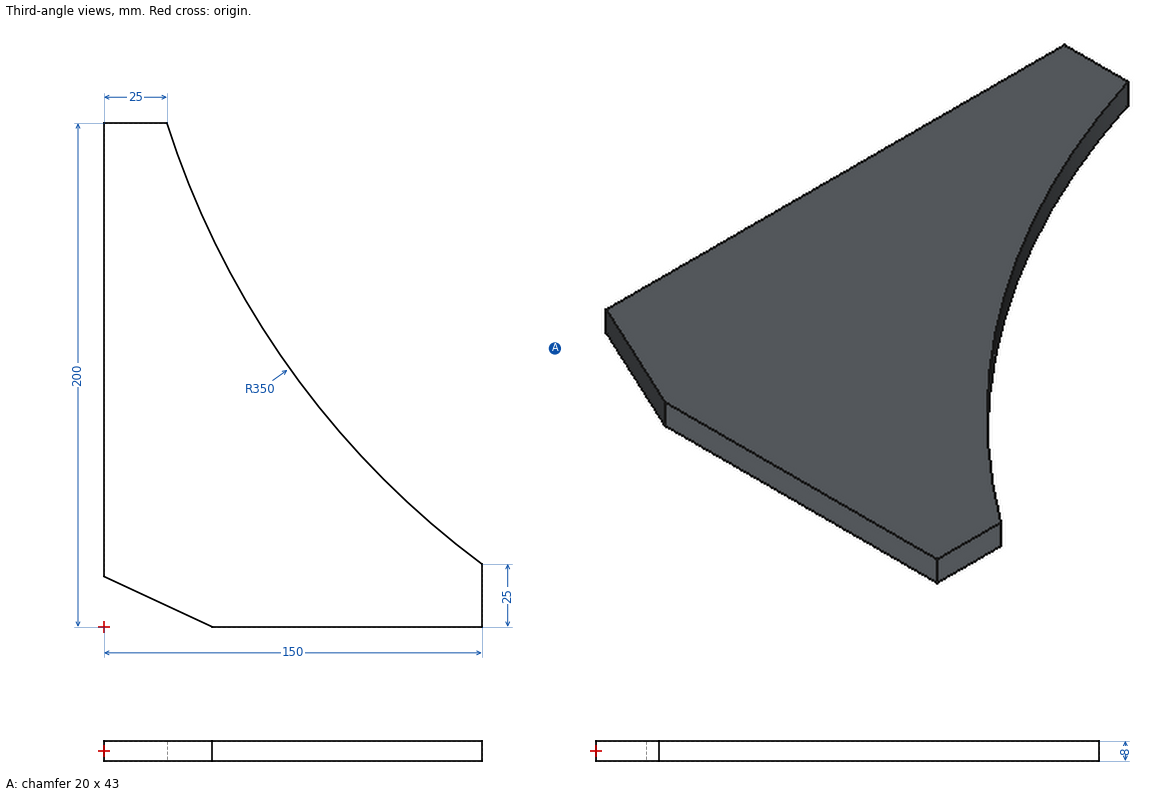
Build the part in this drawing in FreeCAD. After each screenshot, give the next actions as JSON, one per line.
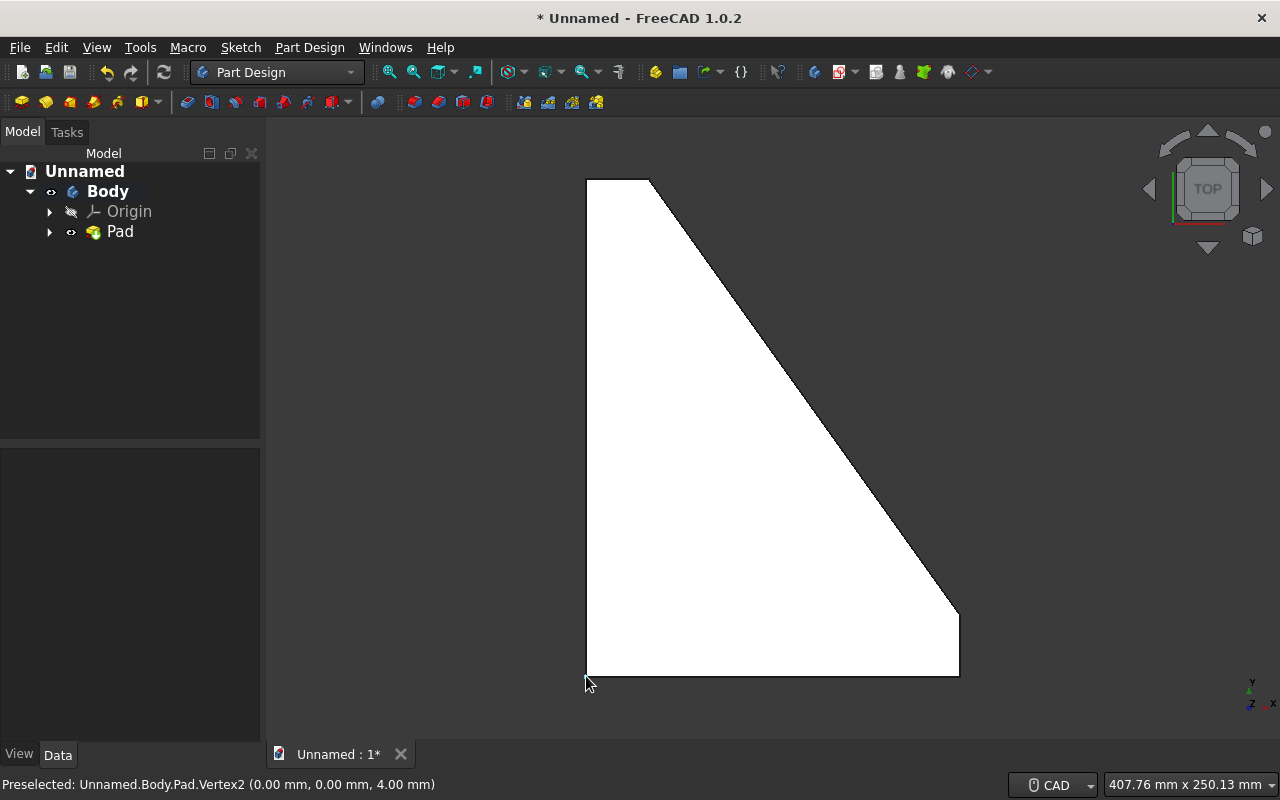
{"action": "key", "text": "1"}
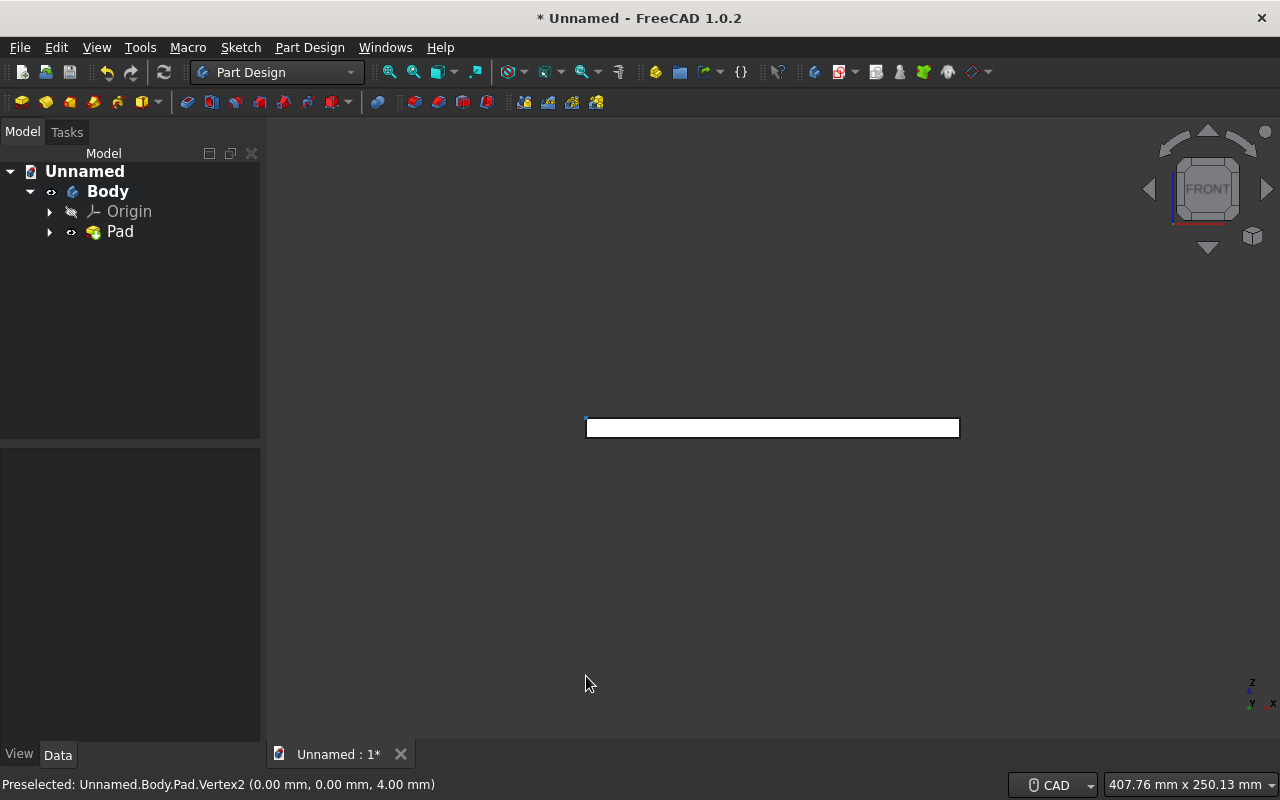
{"action": "left_click", "coordinate": [390, 72]}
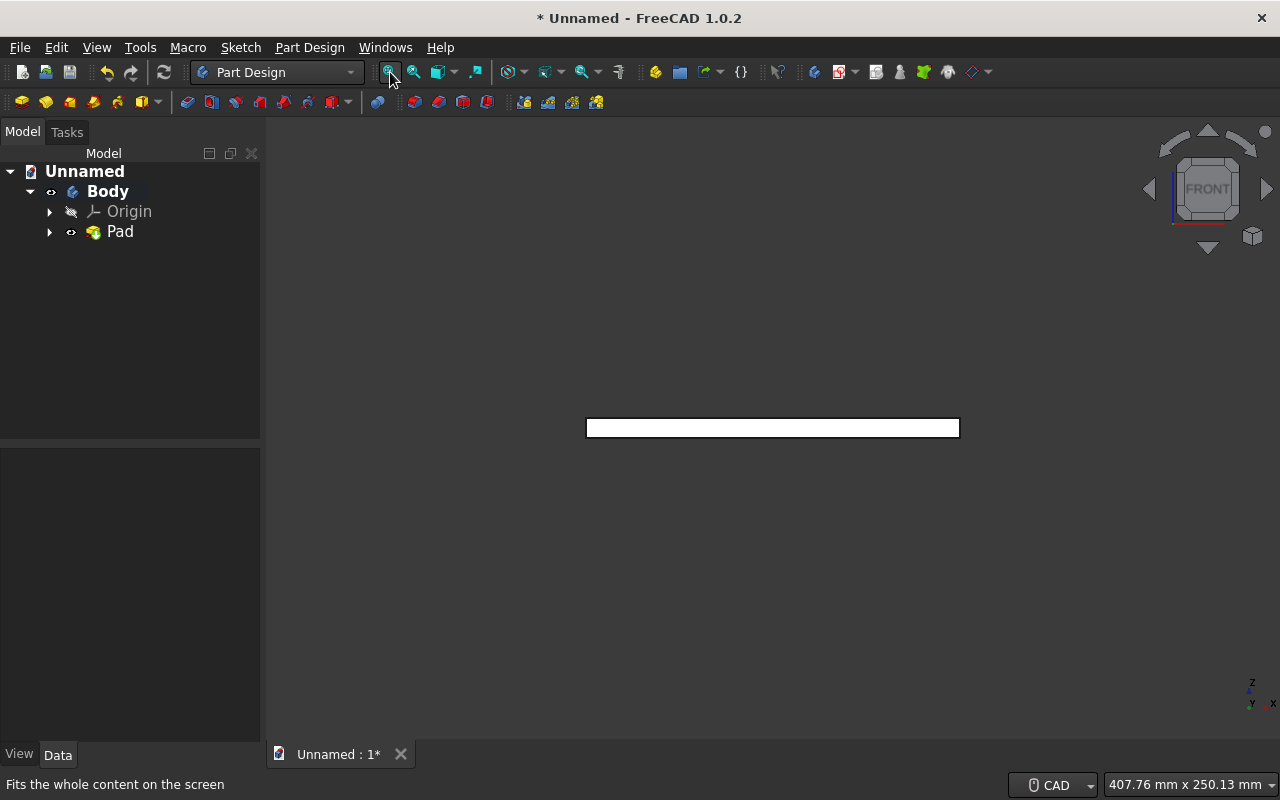
{"action": "left_click", "coordinate": [586, 427]}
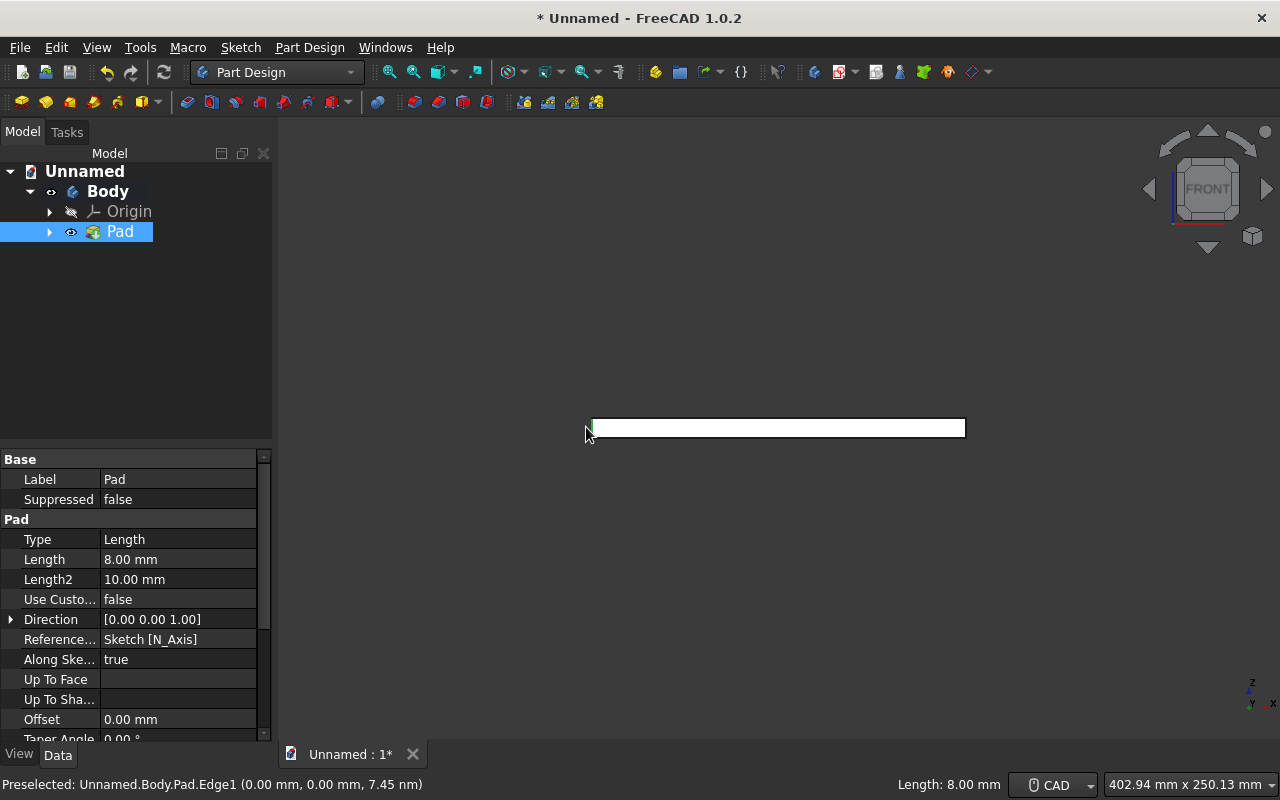
{"action": "left_click", "coordinate": [440, 102]}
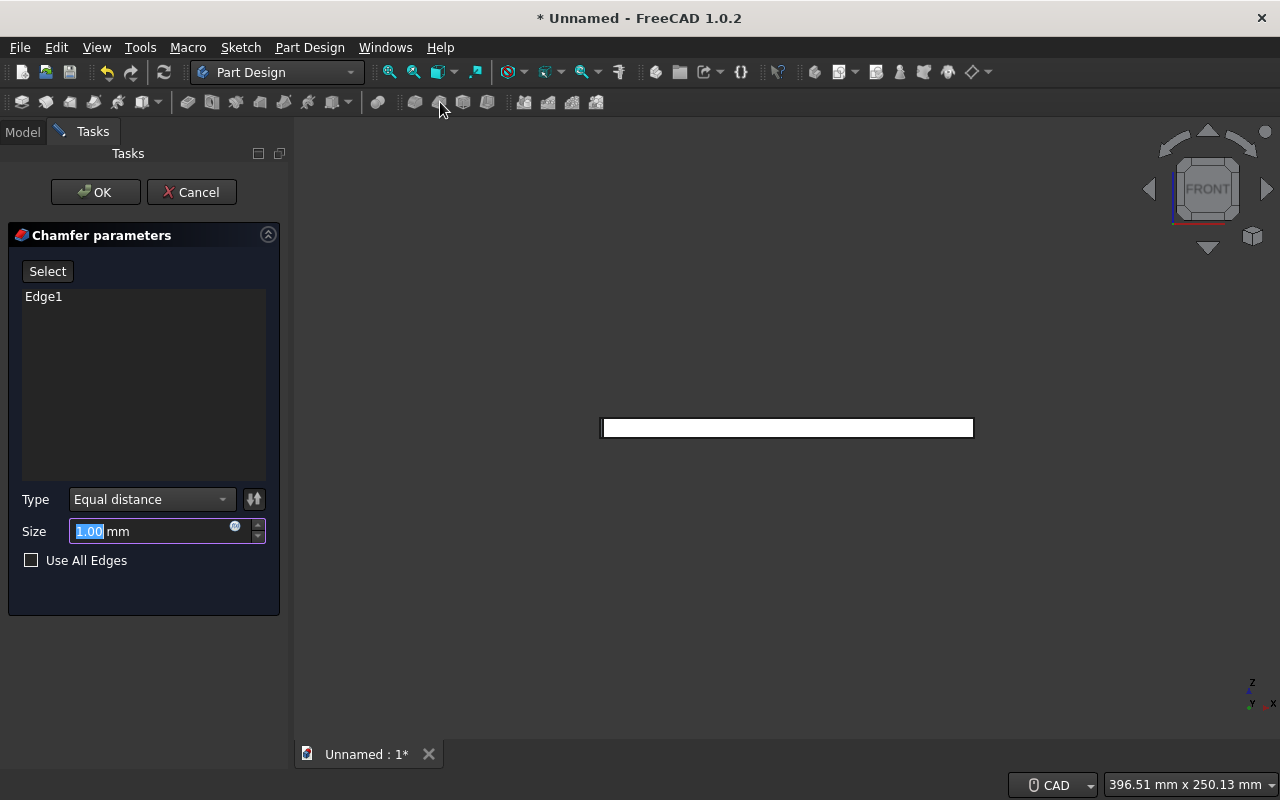
{"action": "type", "text": "20"}
{"action": "key", "text": "Tab"}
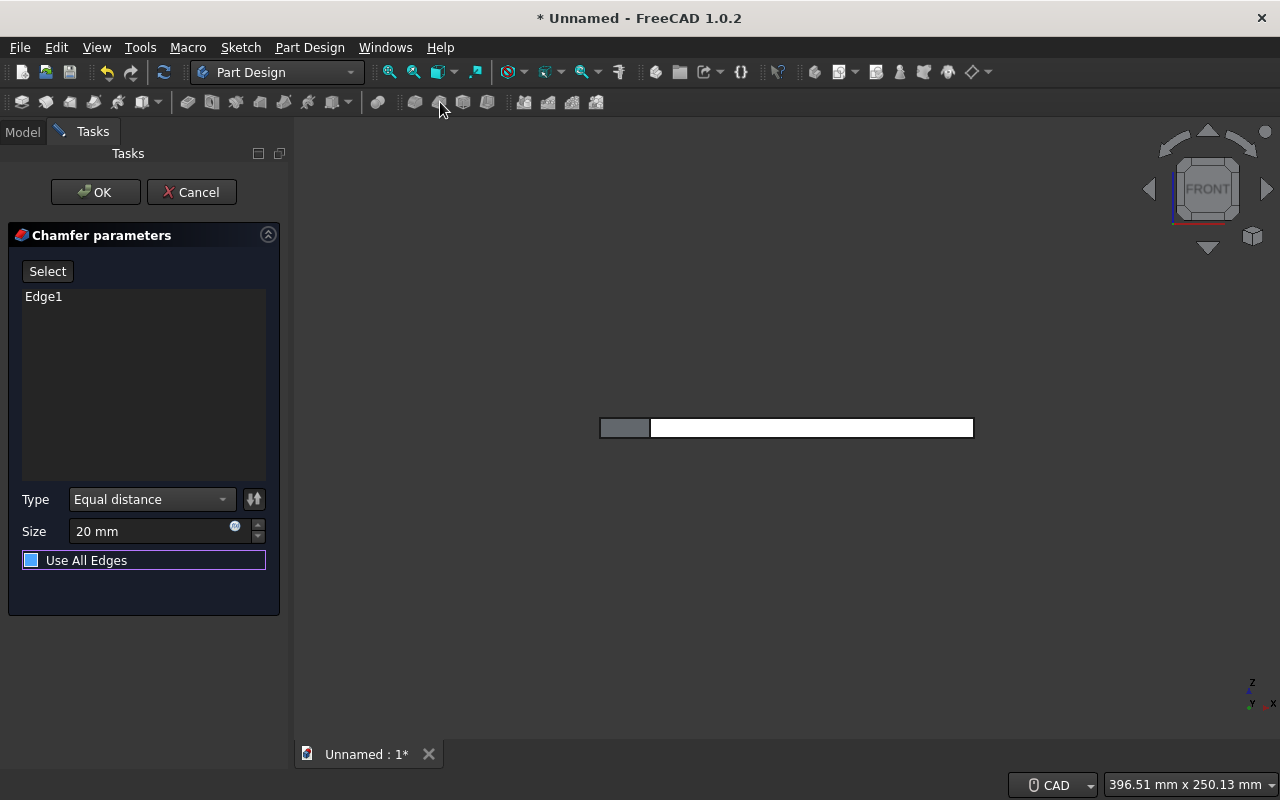
{"action": "left_click", "coordinate": [153, 500]}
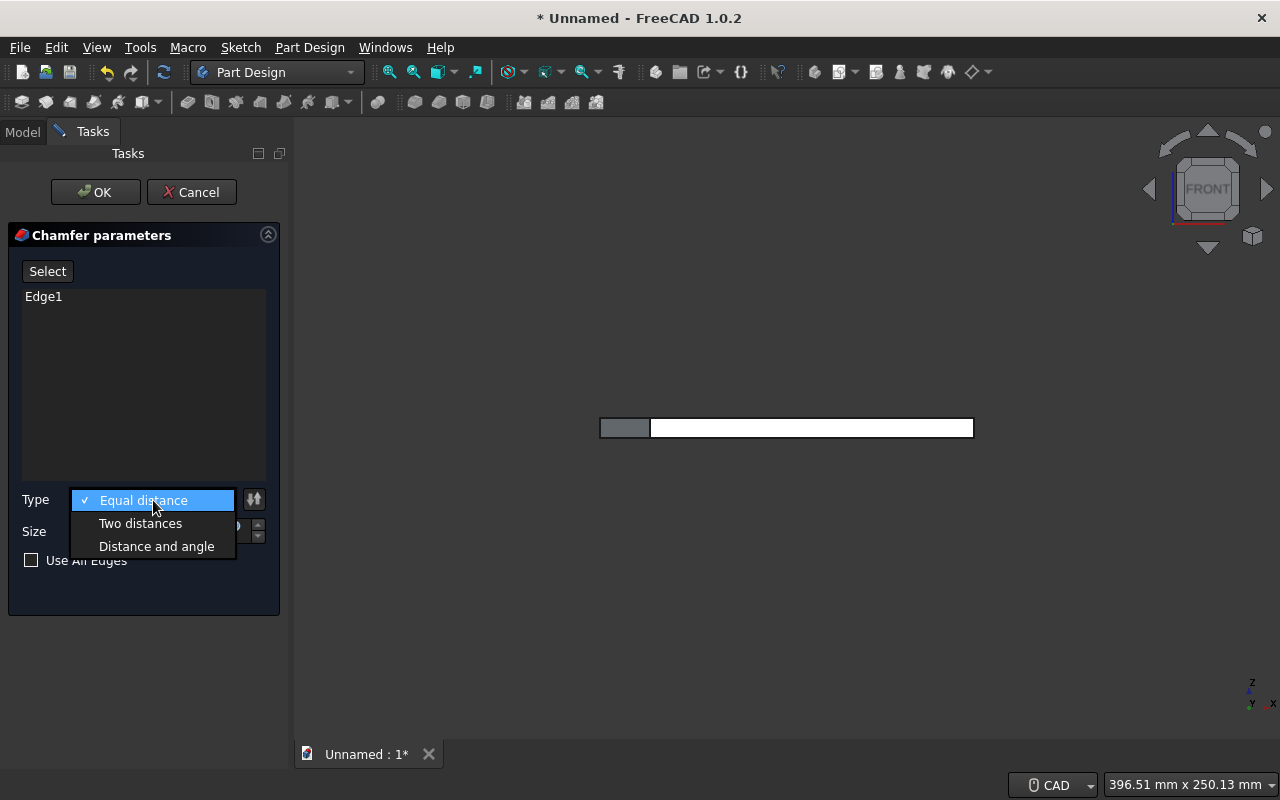
{"action": "left_click", "coordinate": [152, 524]}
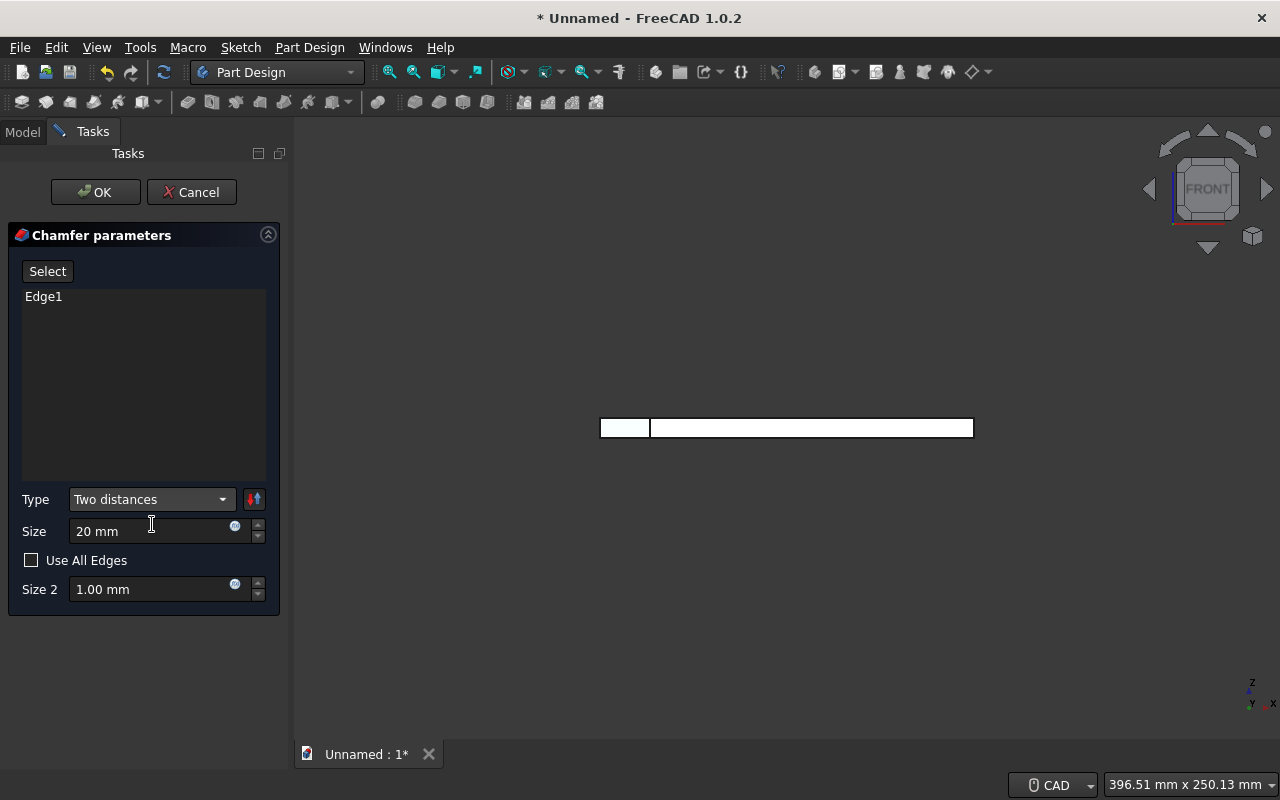
{"action": "triple_click", "coordinate": [160, 589]}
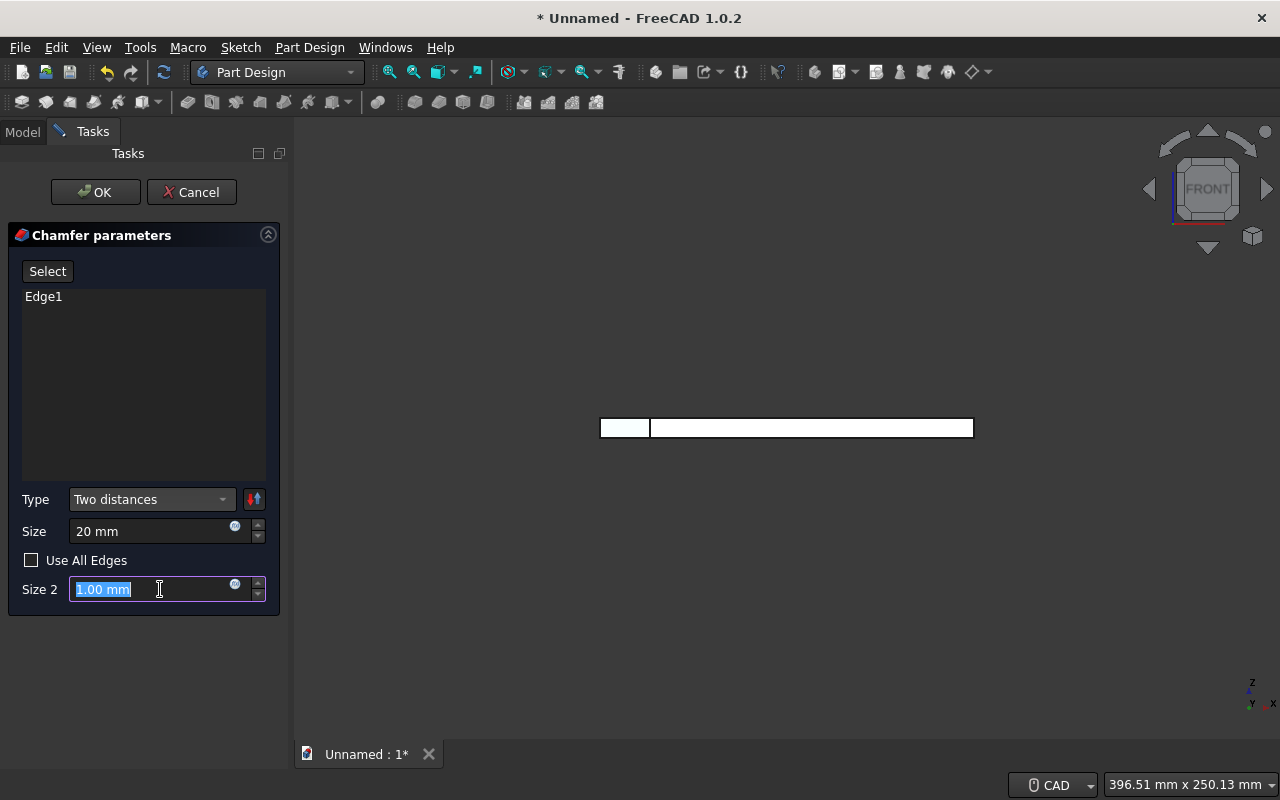
{"action": "type", "text": "43"}
{"action": "key", "text": "Tab"}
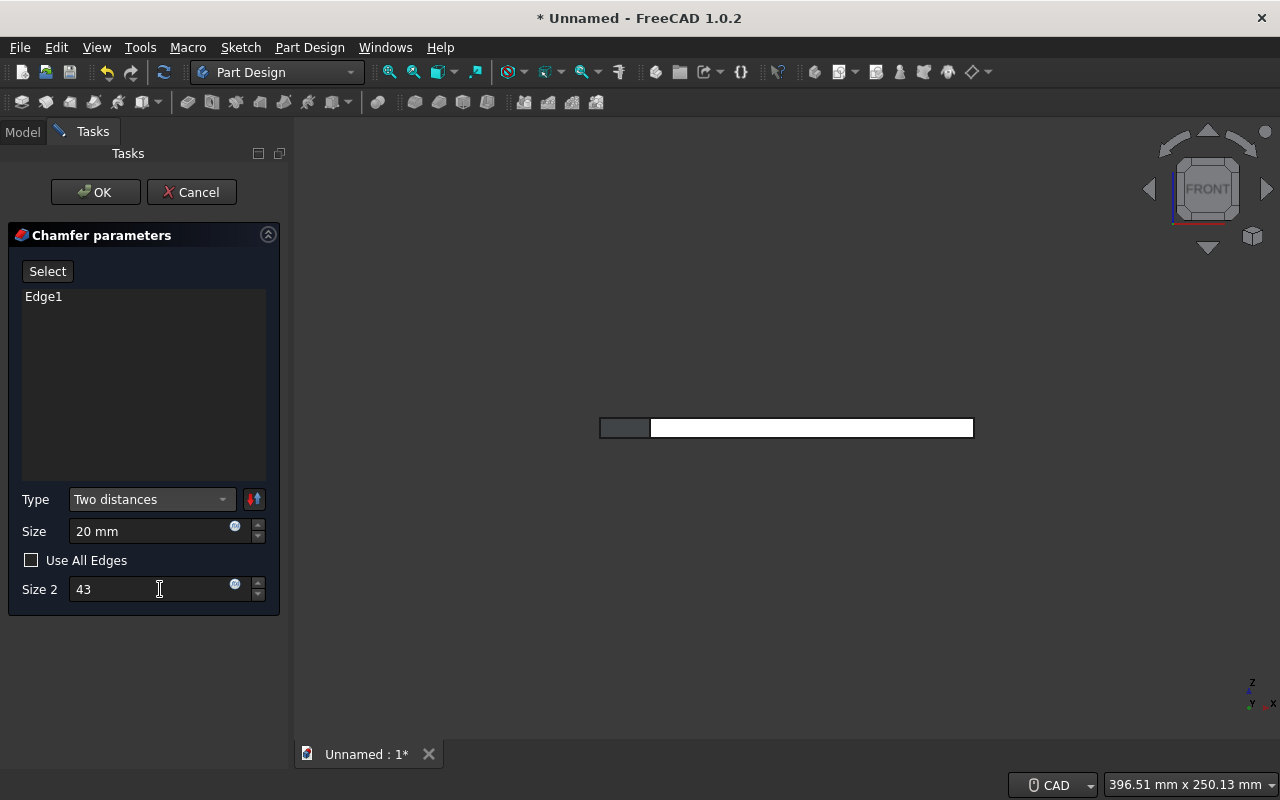
{"action": "left_click", "coordinate": [254, 500]}